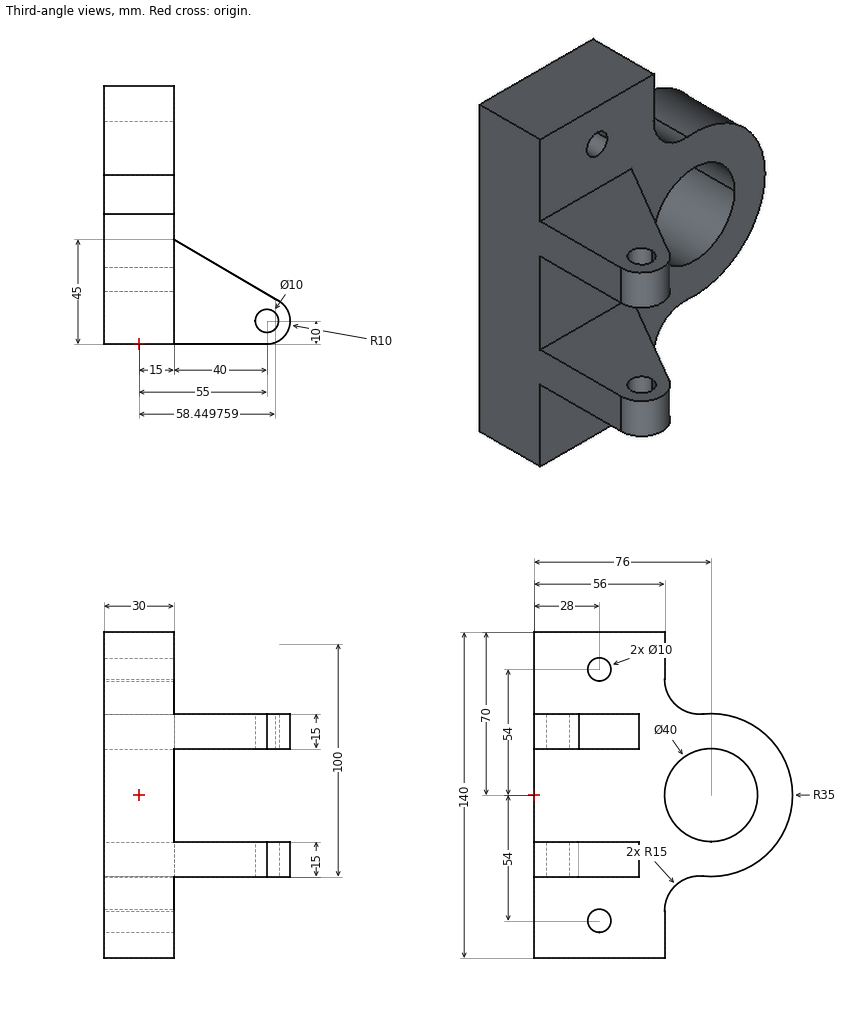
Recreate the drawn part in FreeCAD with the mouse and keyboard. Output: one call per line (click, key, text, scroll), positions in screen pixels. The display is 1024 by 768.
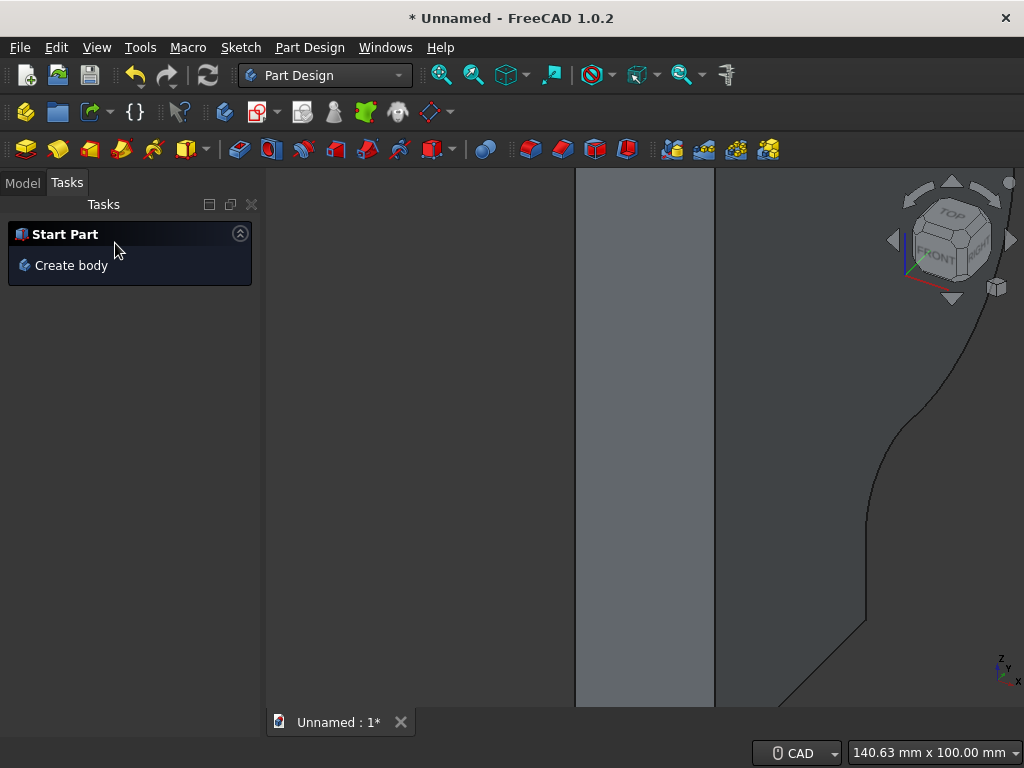
key(v)
key(f)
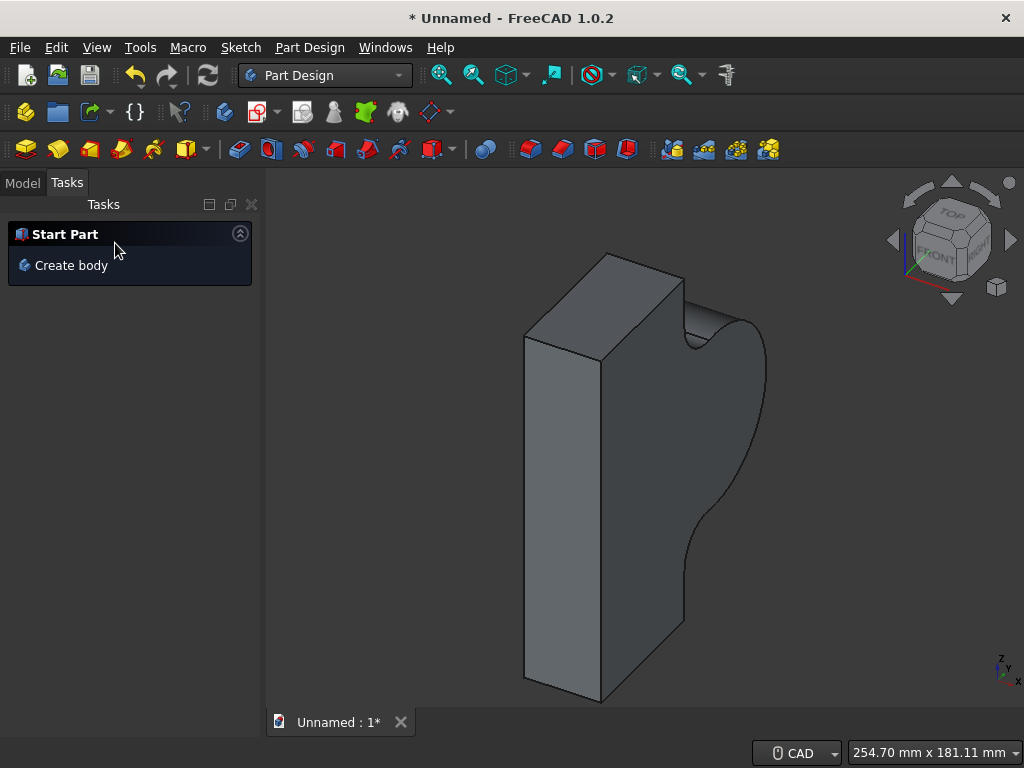
click(23, 182)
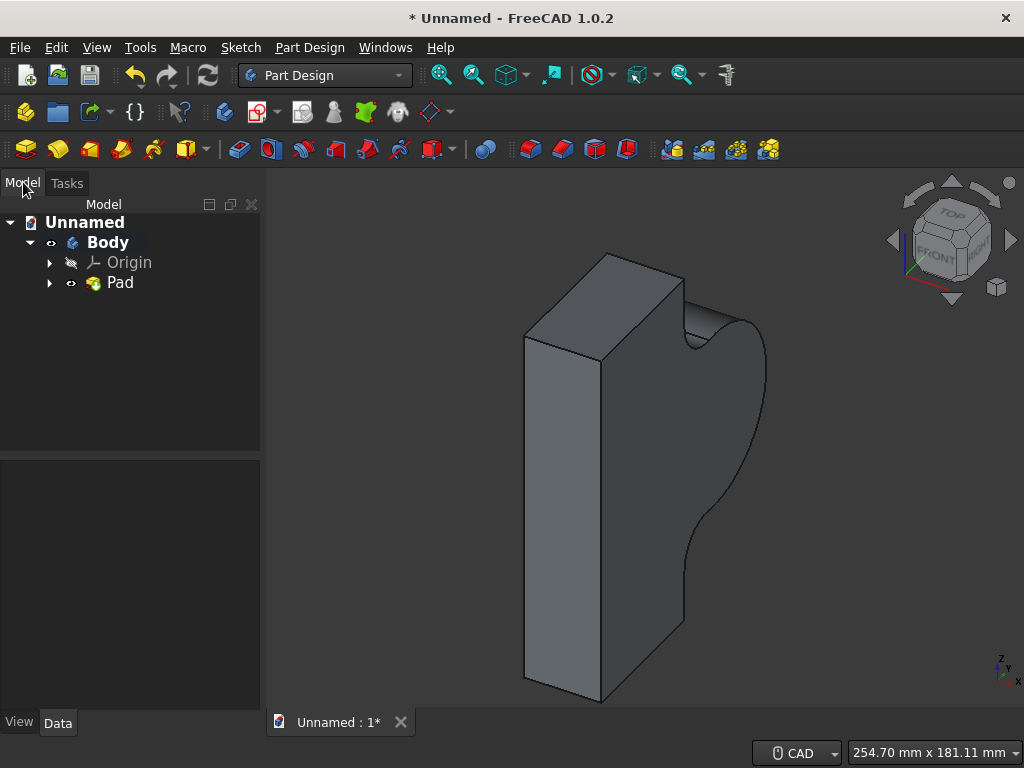
click(50, 263)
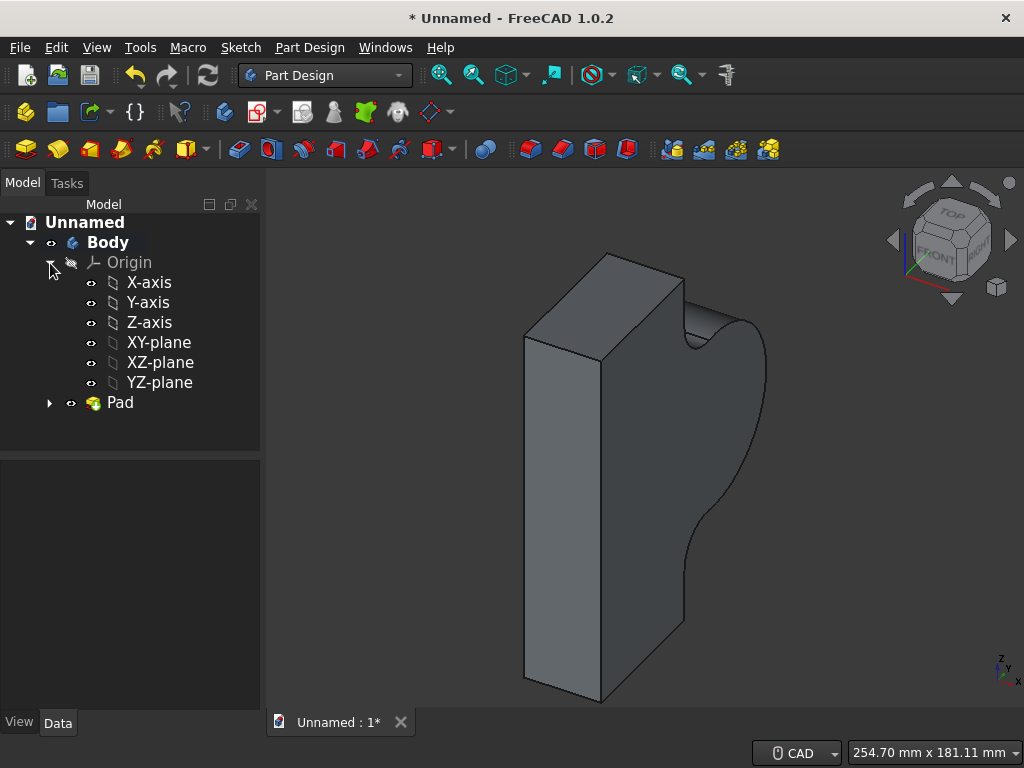
click(136, 343)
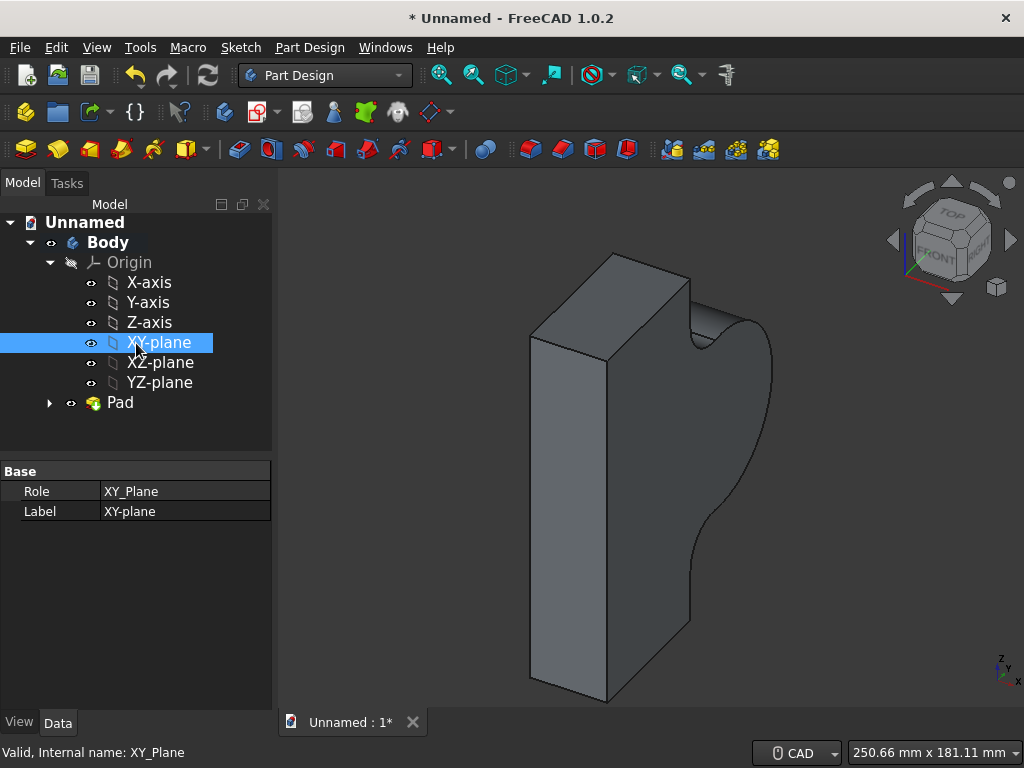
click(430, 112)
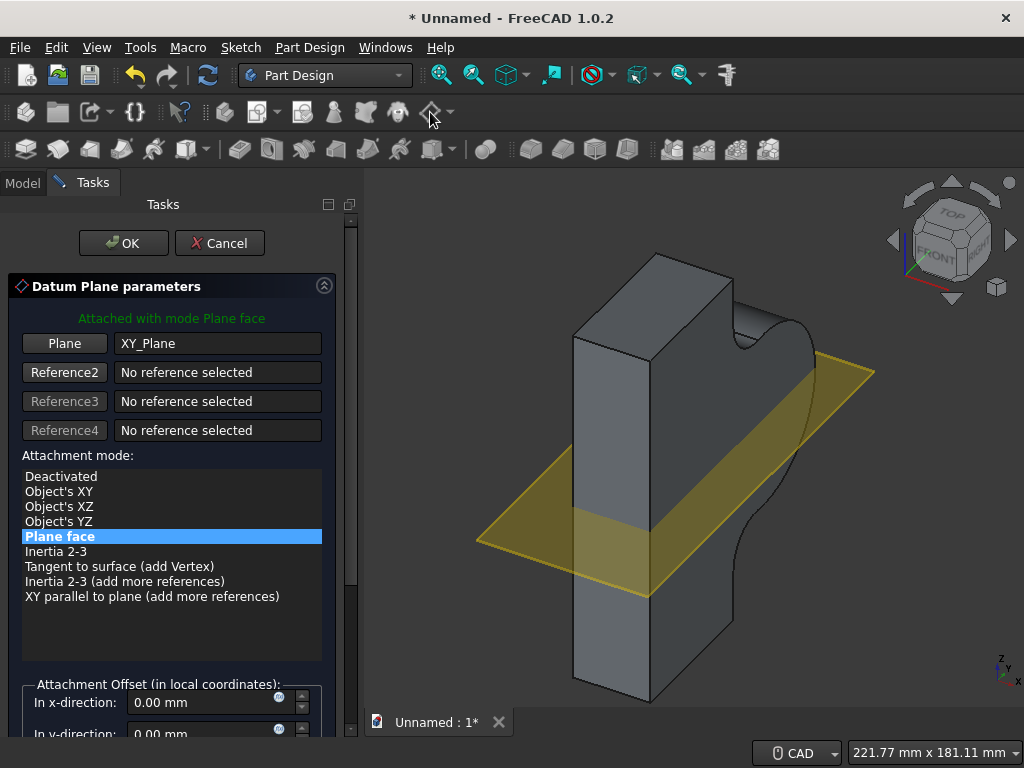
scroll(351, 475, down, 2)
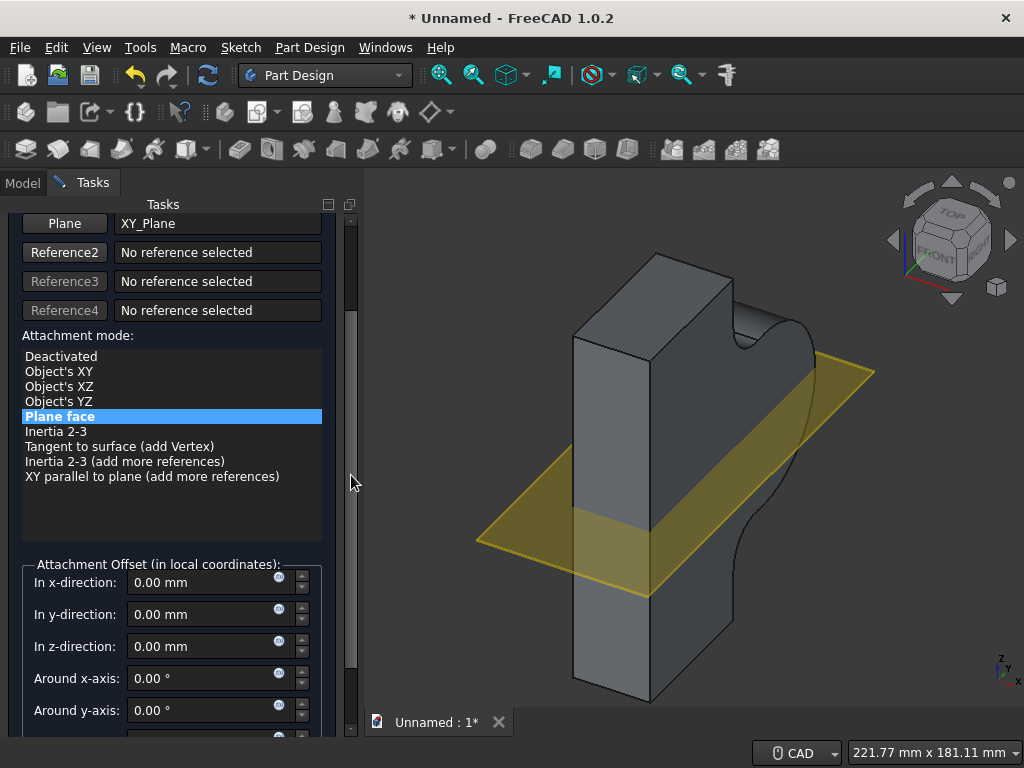
triple_click(210, 646)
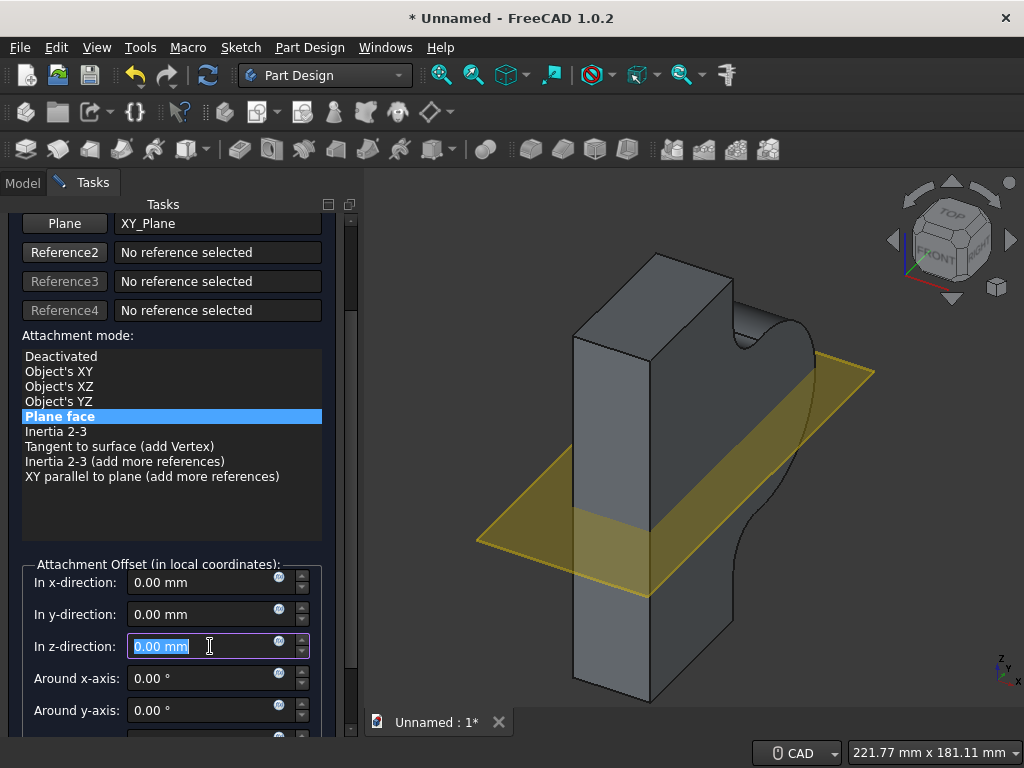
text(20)
key(Tab)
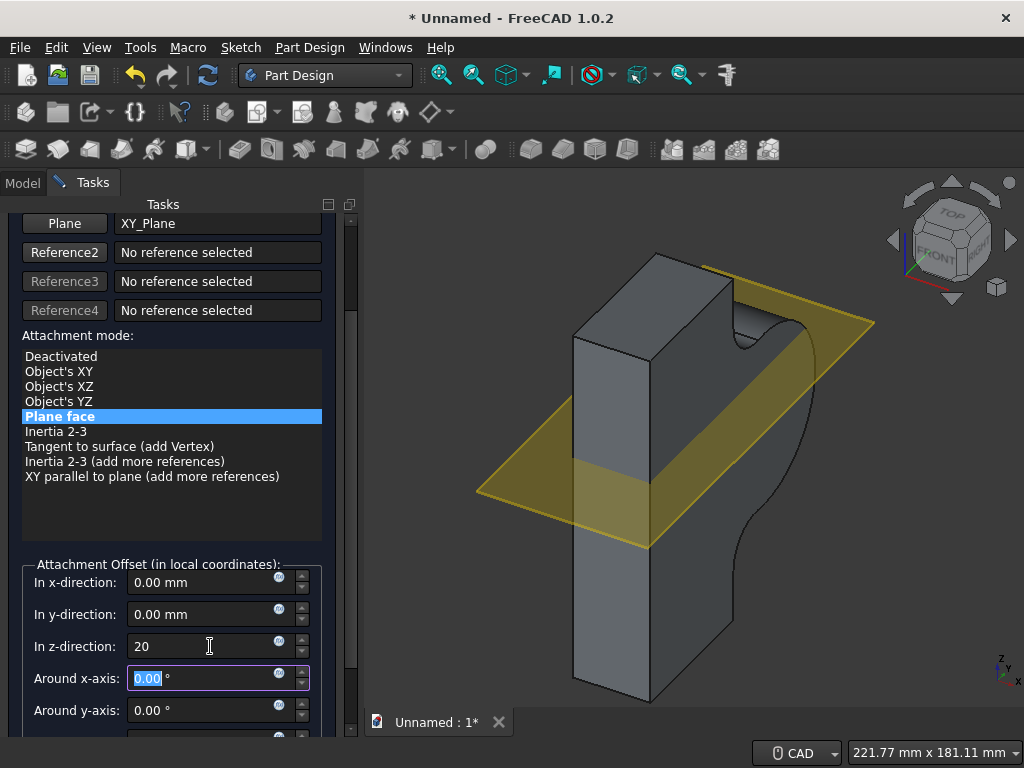
scroll(351, 475, up, 3)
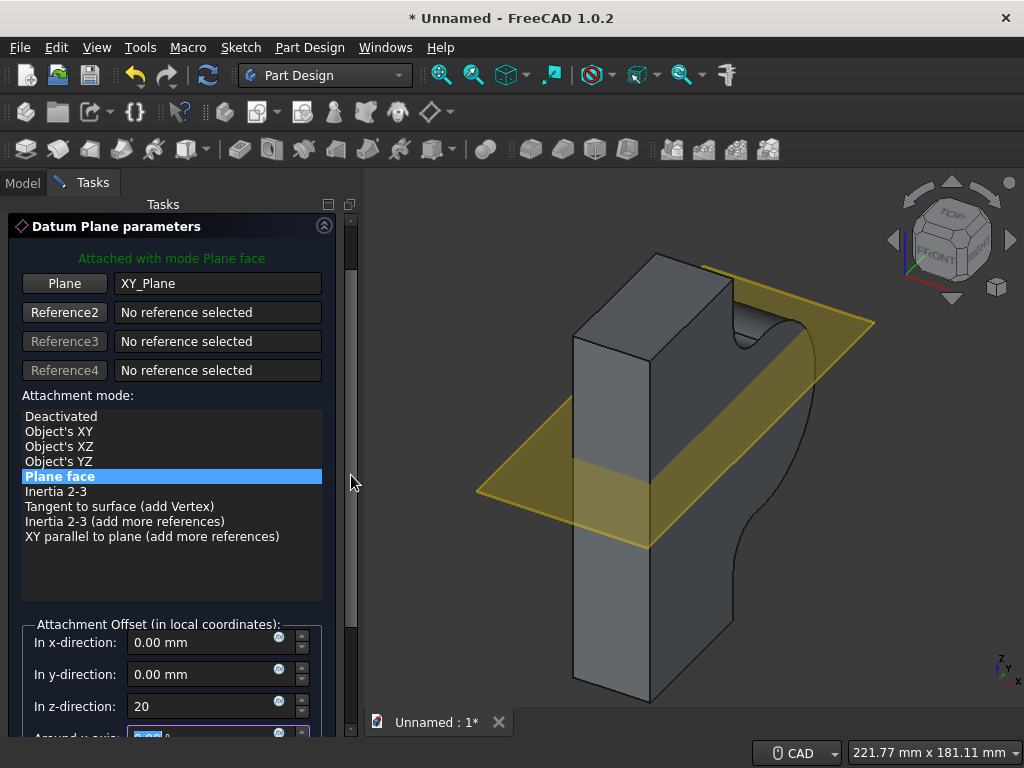
click(124, 243)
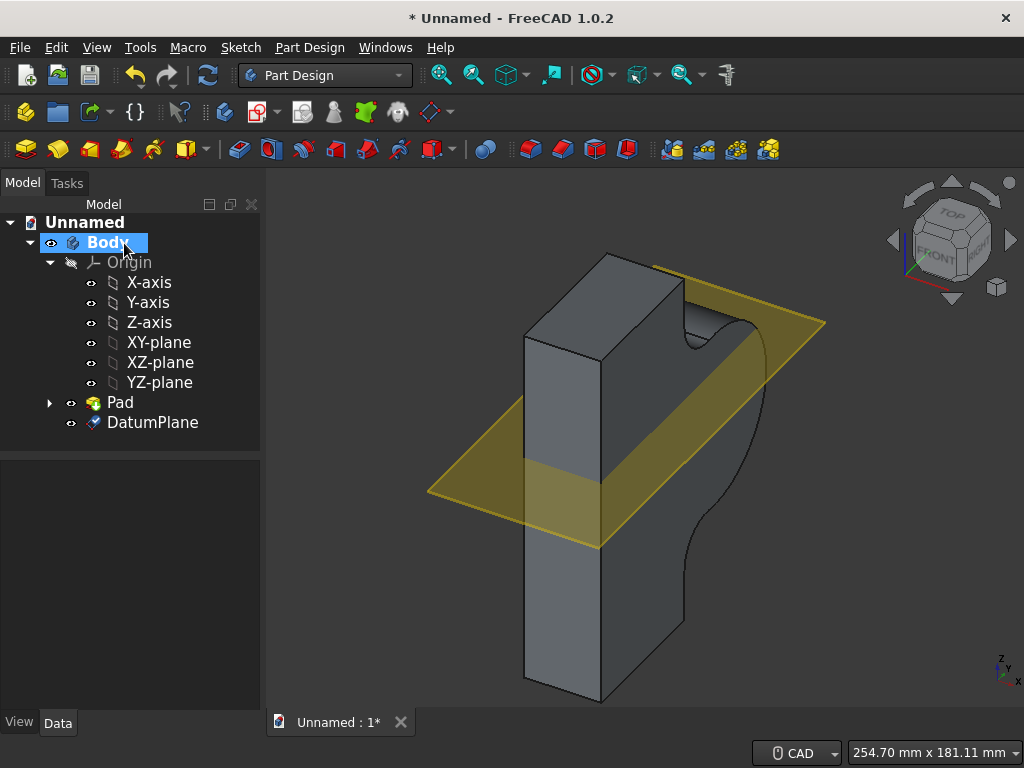
click(116, 423)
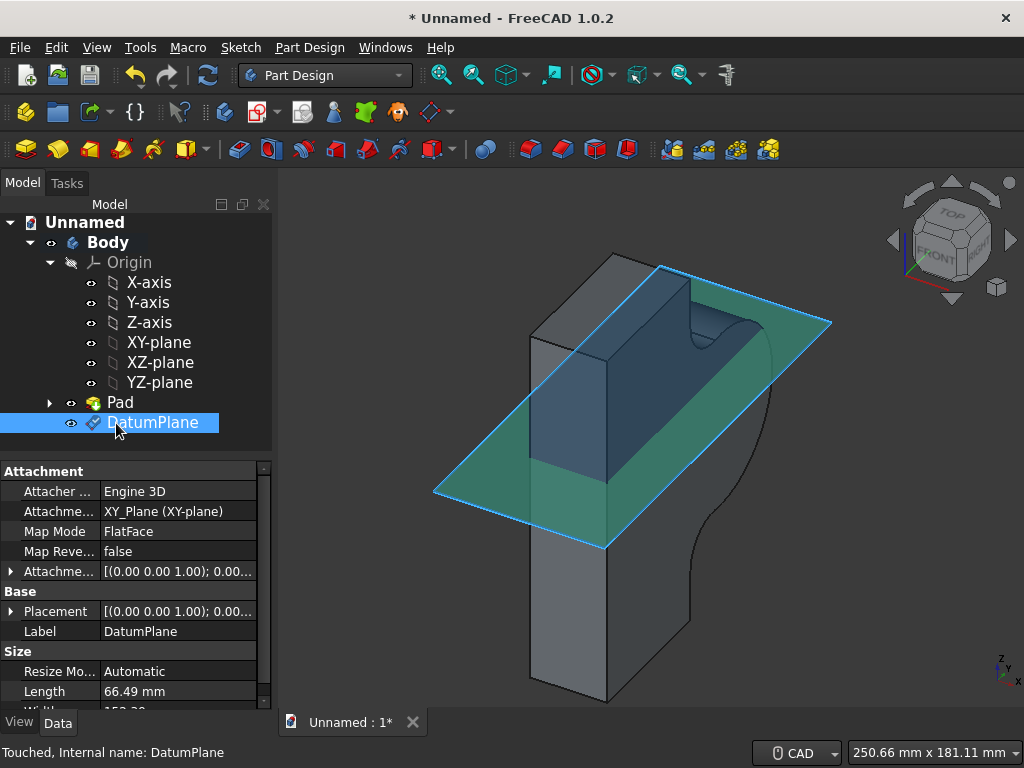
click(258, 112)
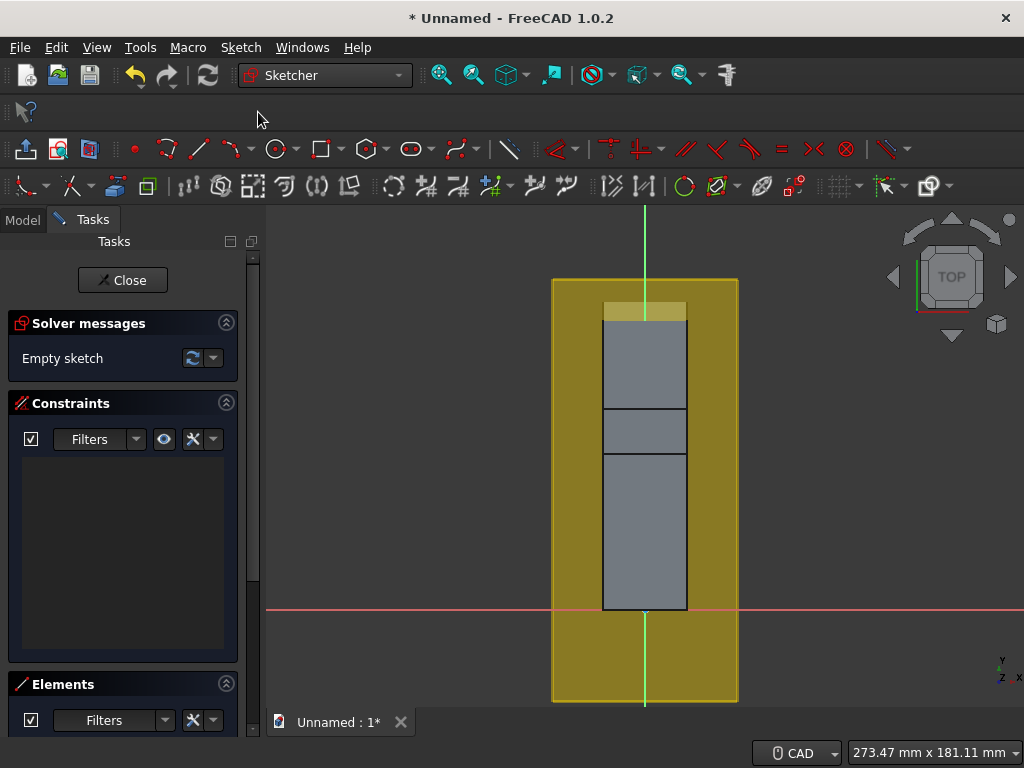
key(q)
key(s)